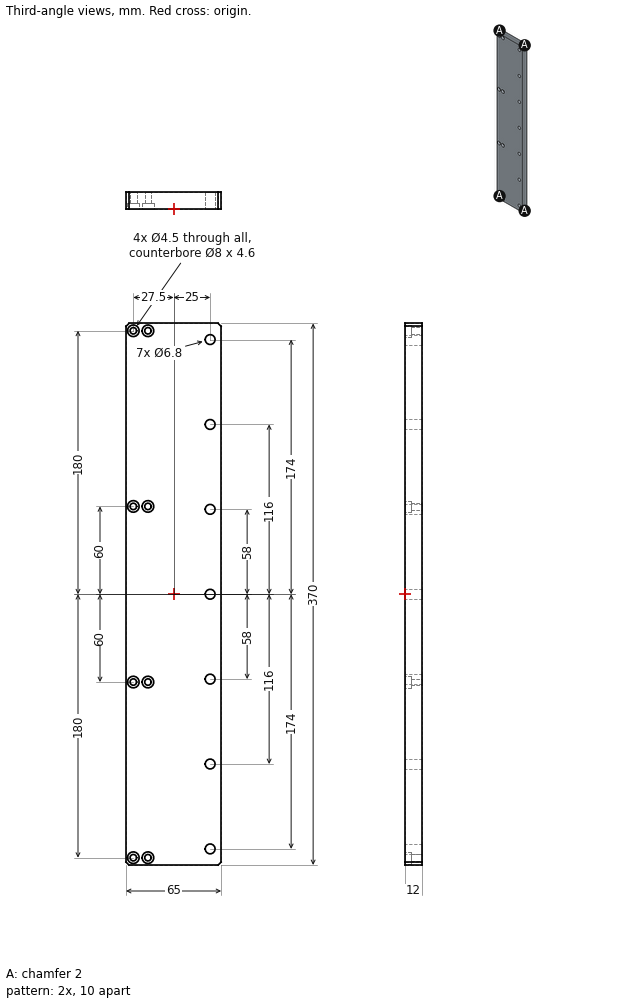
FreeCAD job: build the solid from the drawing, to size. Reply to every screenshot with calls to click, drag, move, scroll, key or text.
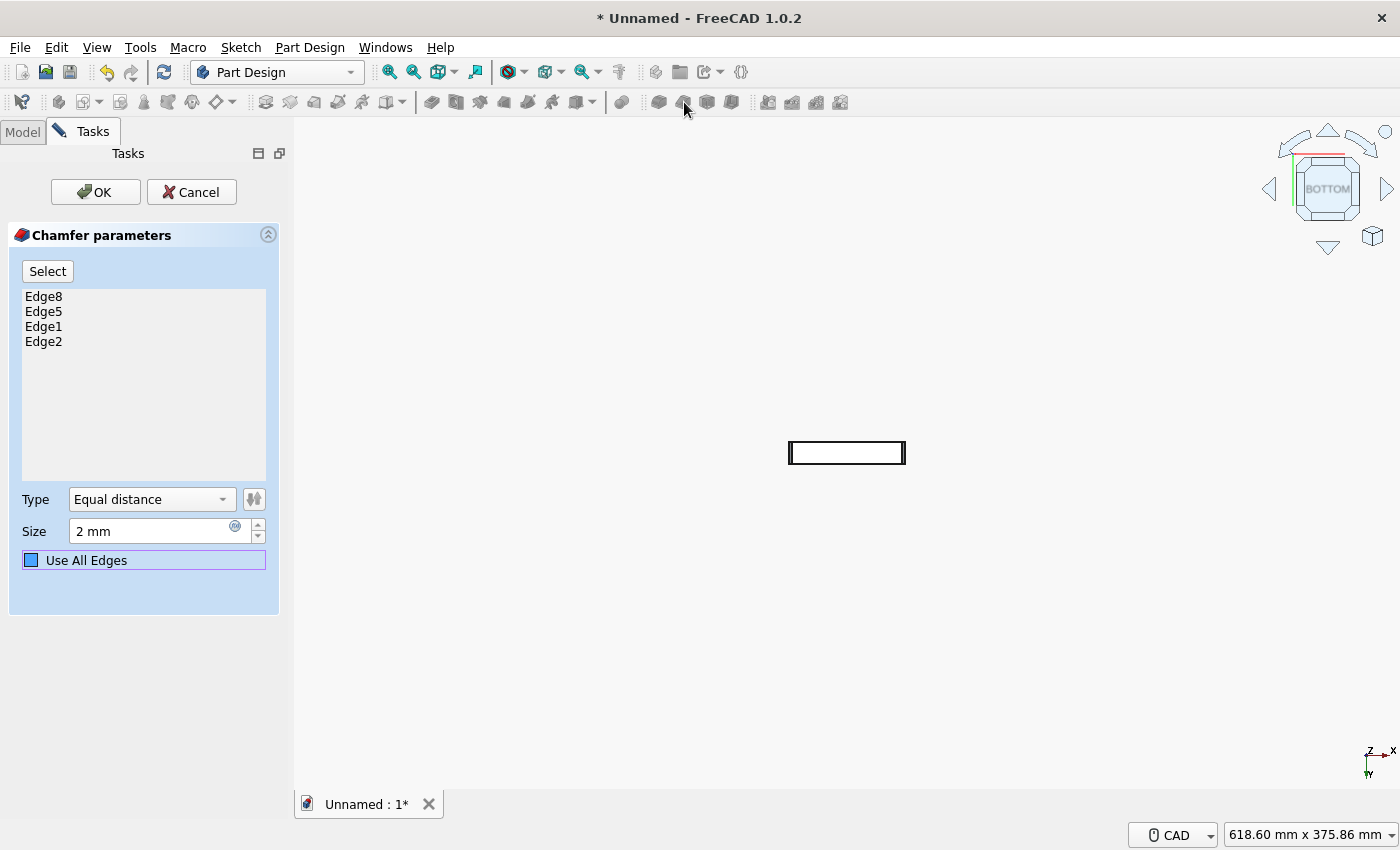
click(96, 192)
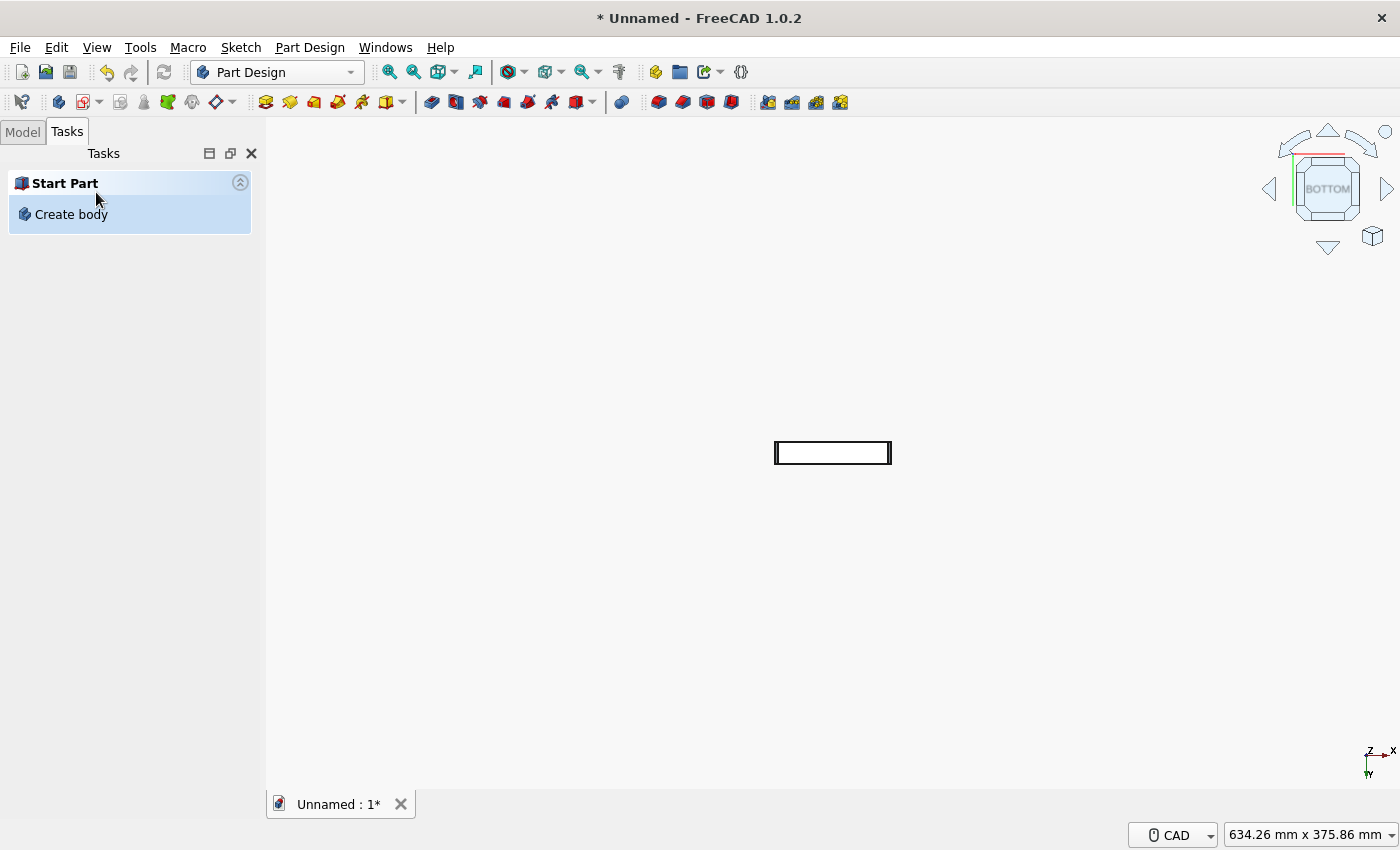
click(390, 72)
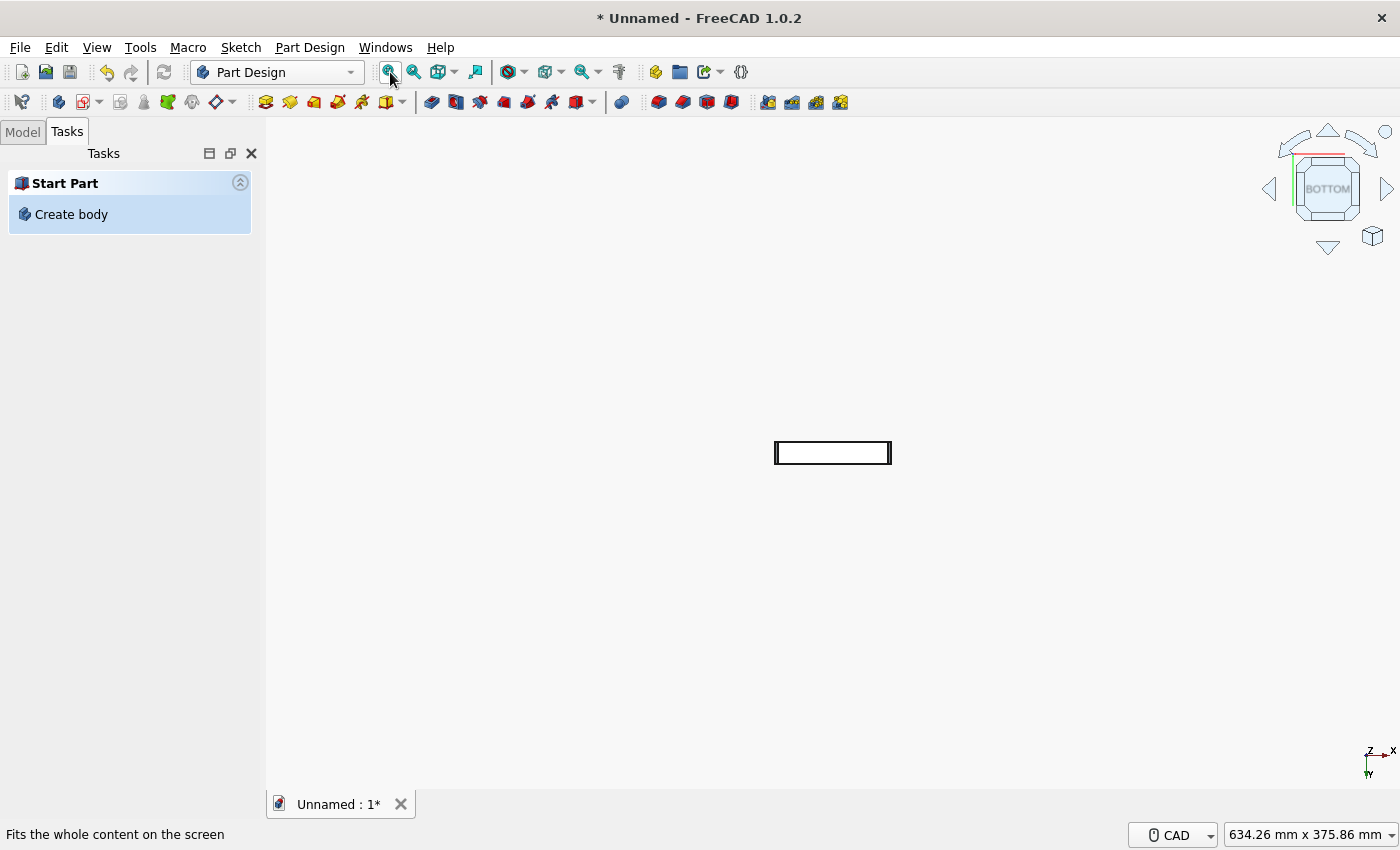
click(23, 131)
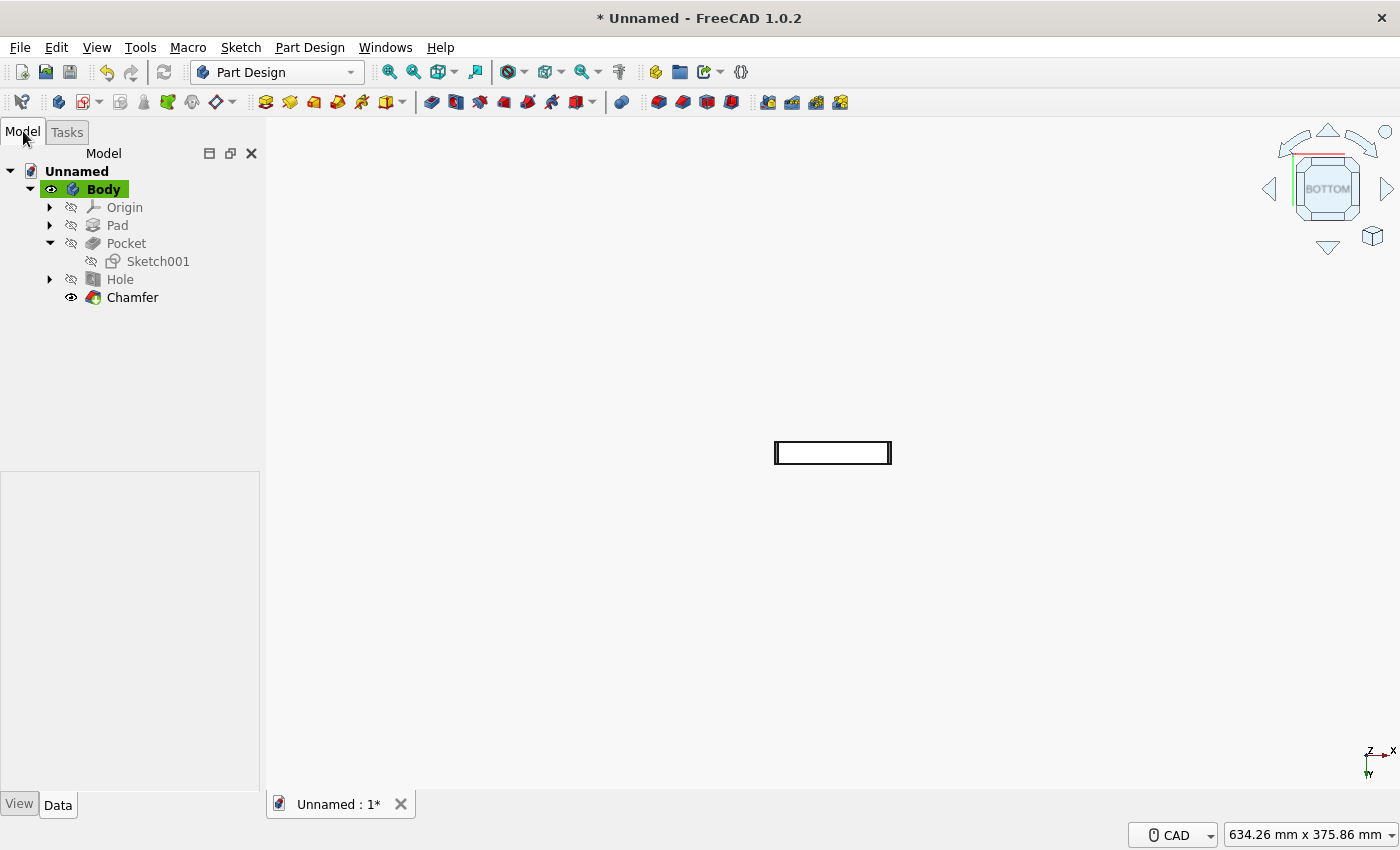
click(116, 279)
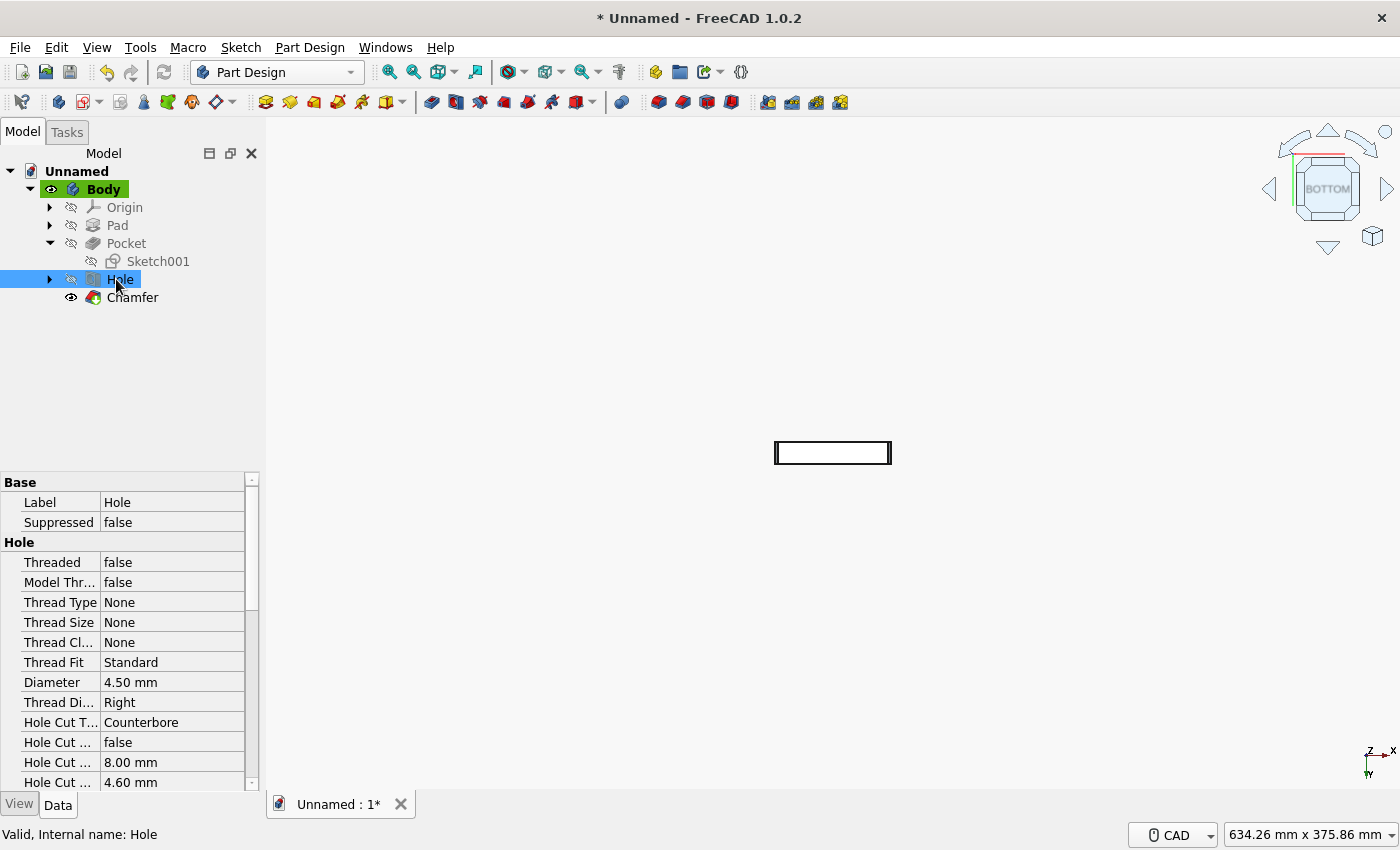
click(792, 102)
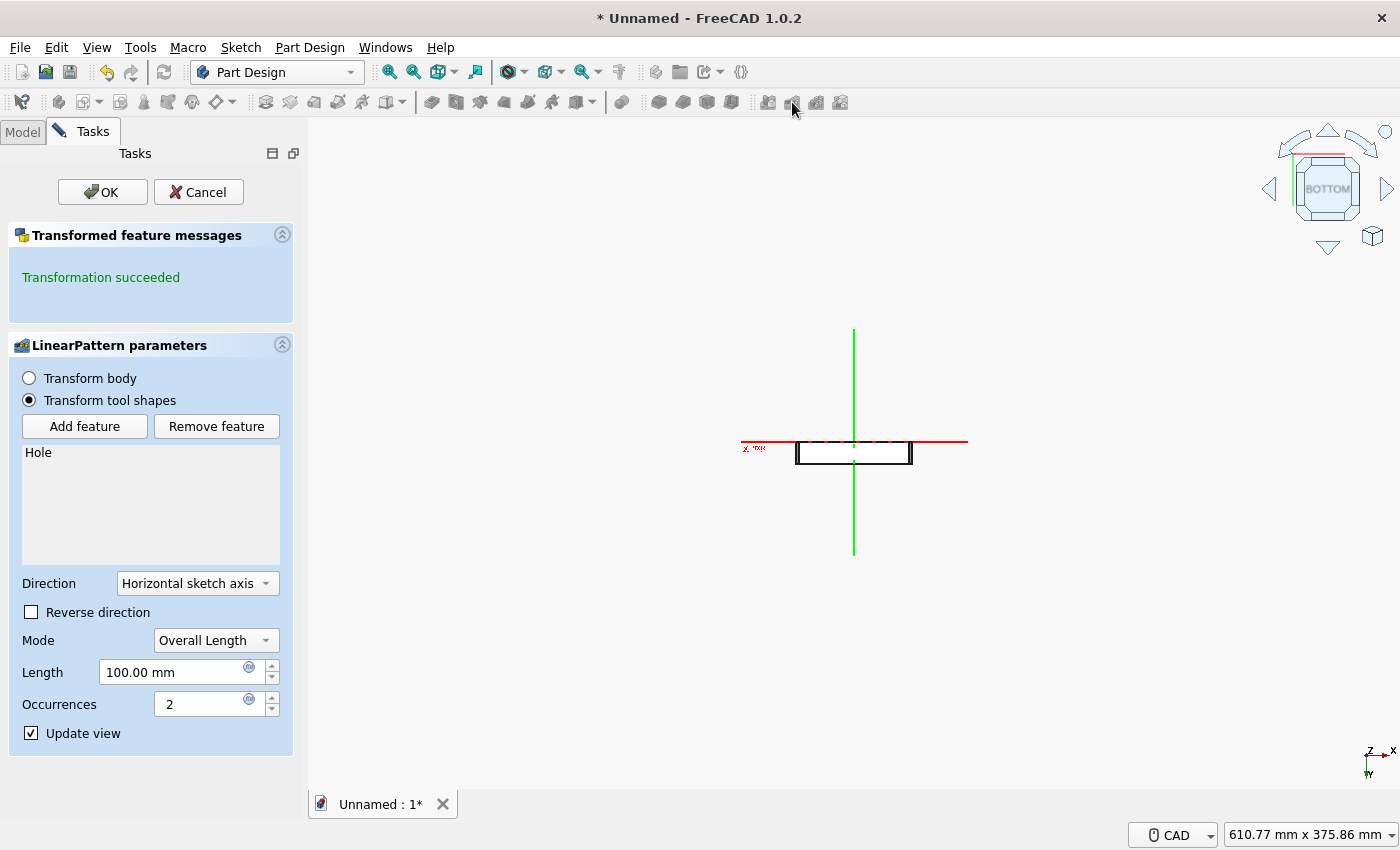
click(198, 584)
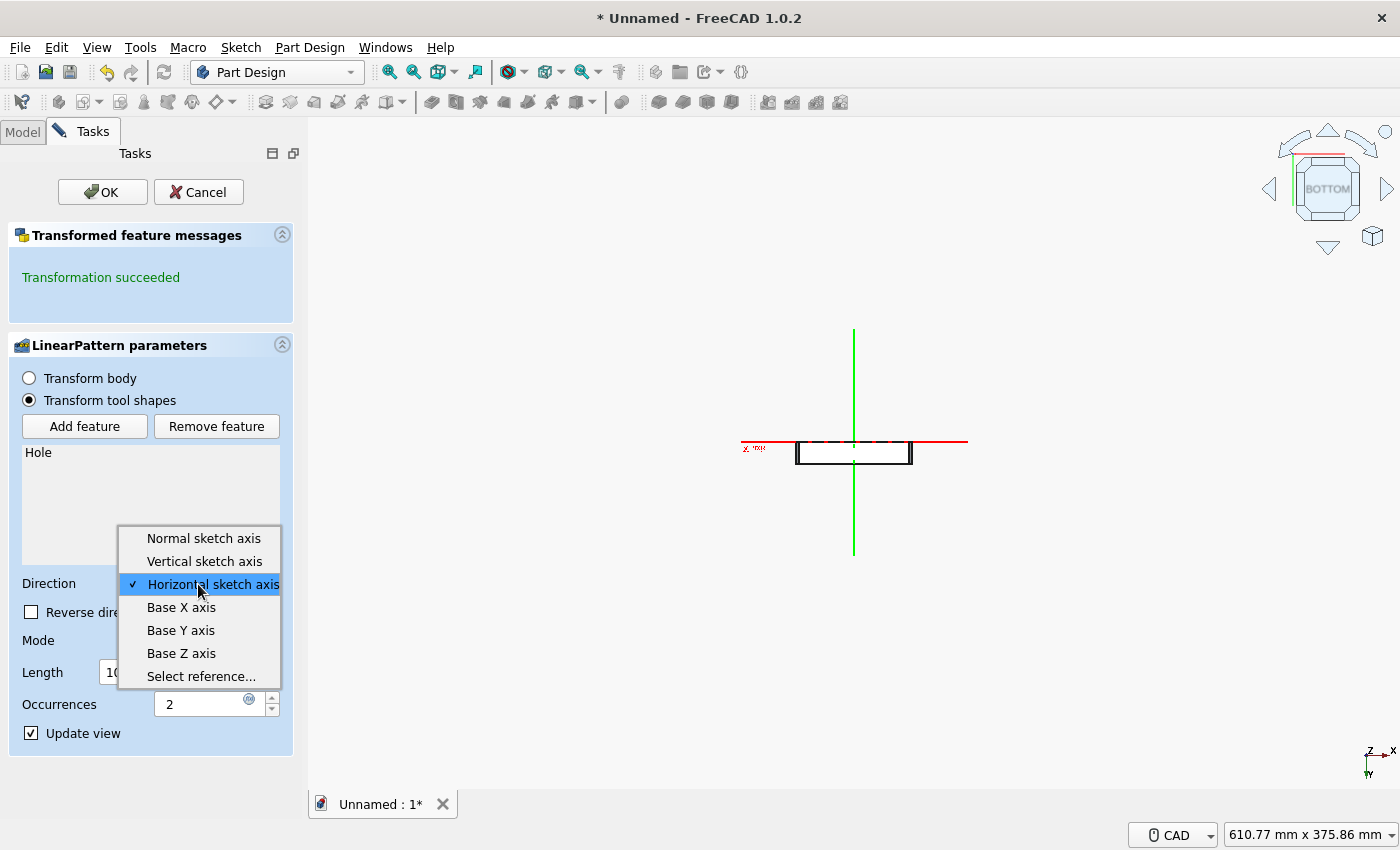
click(198, 608)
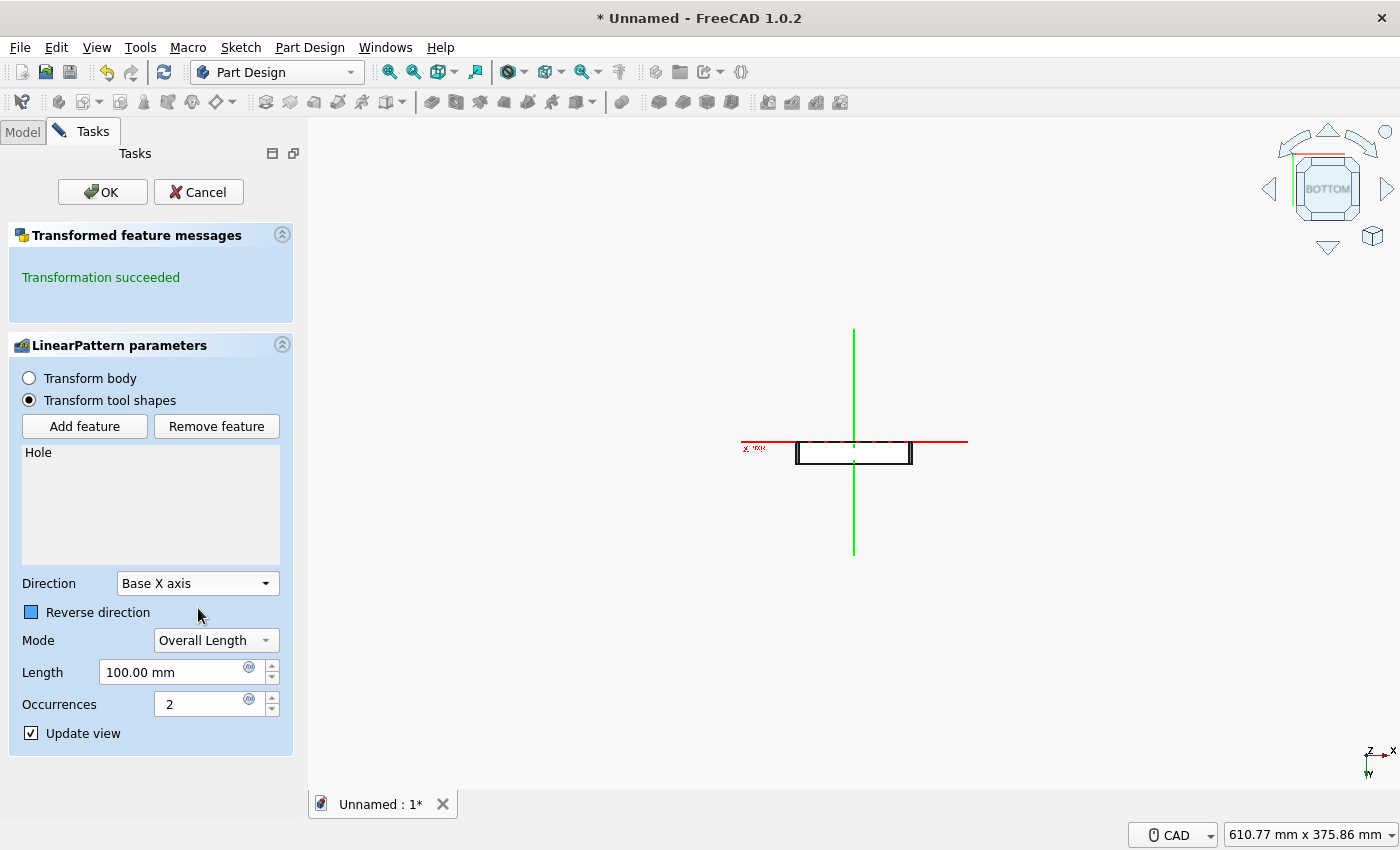
click(217, 640)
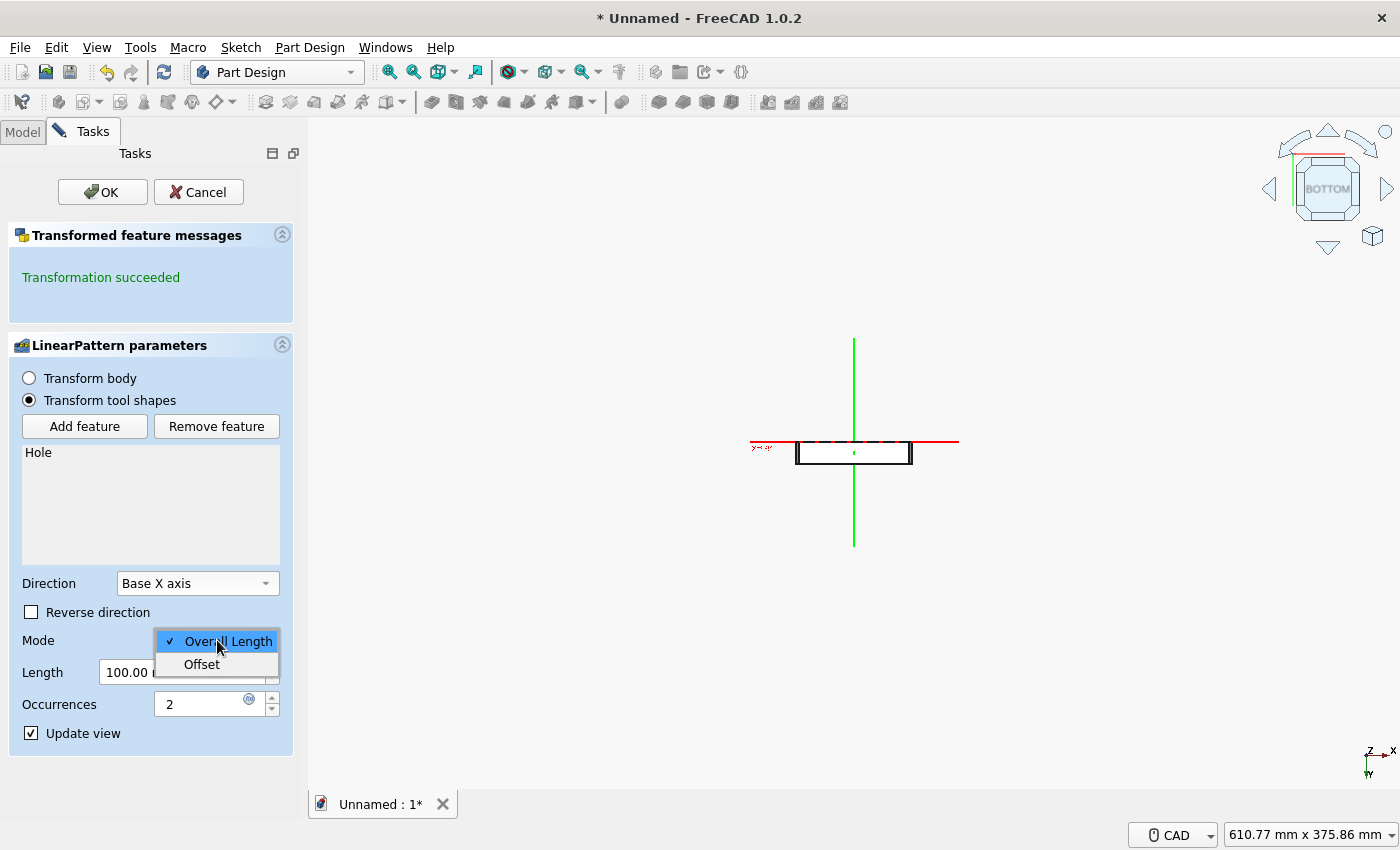
click(216, 664)